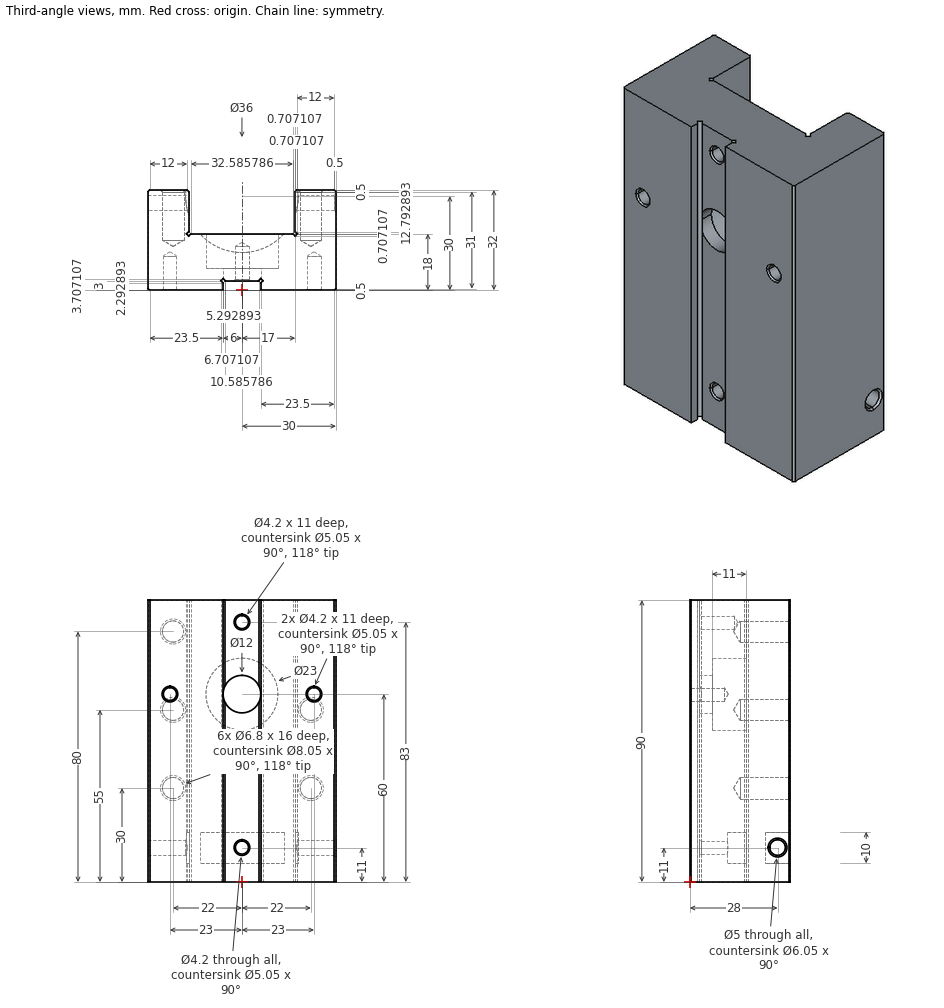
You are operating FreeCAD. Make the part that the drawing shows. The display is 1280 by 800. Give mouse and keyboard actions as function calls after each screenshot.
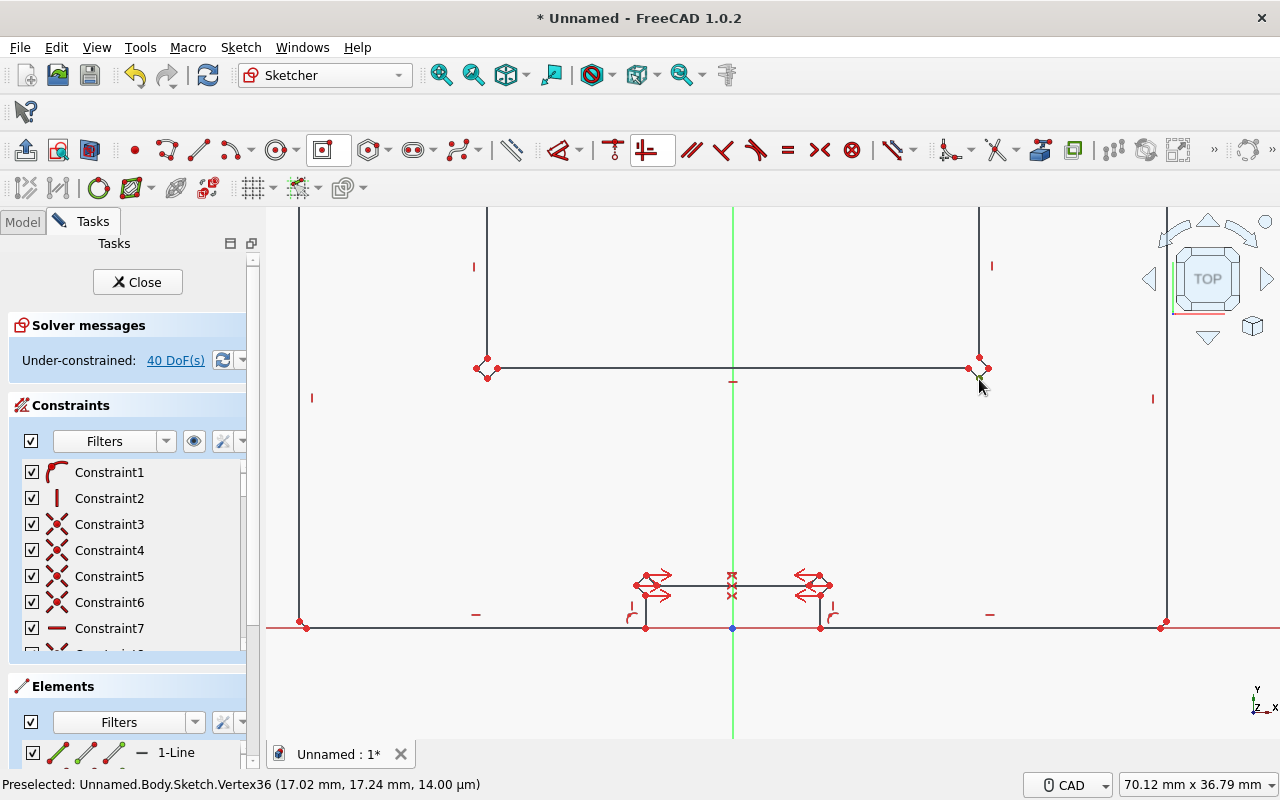
click(487, 379)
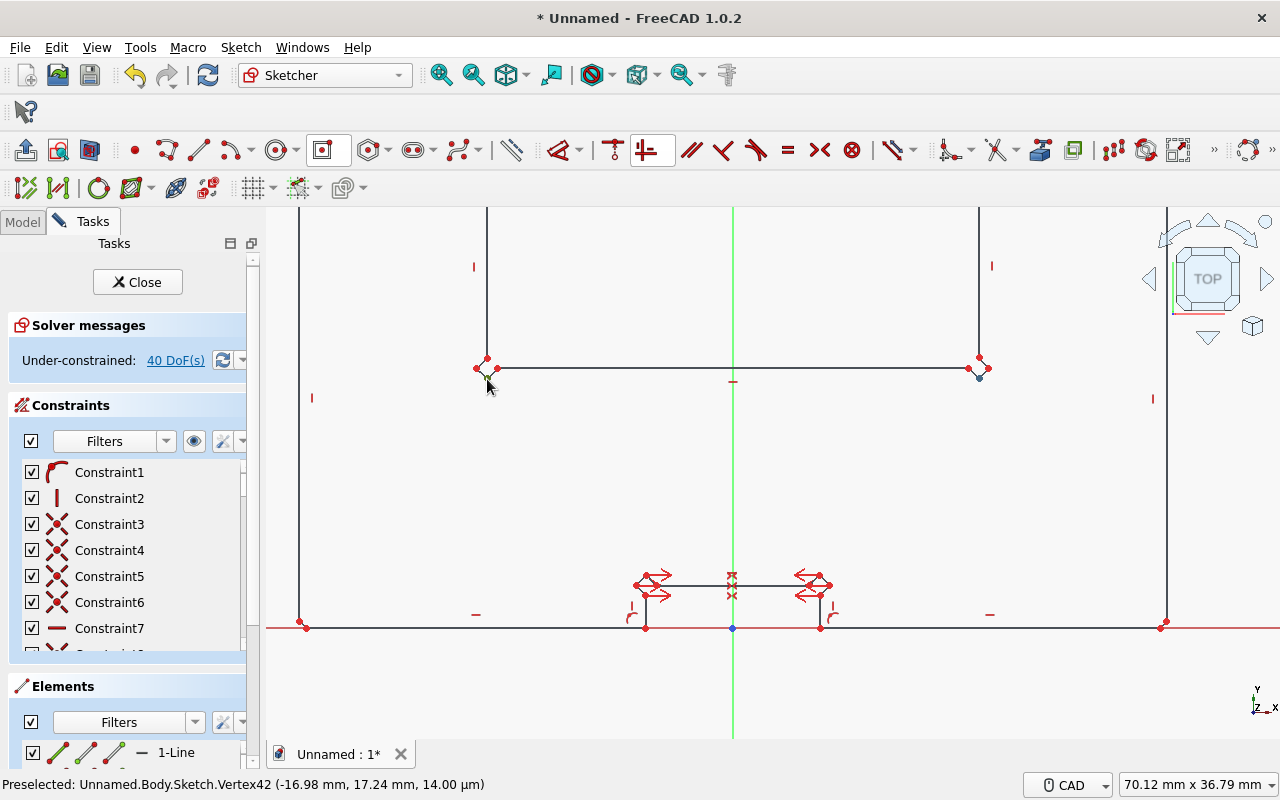
click(733, 677)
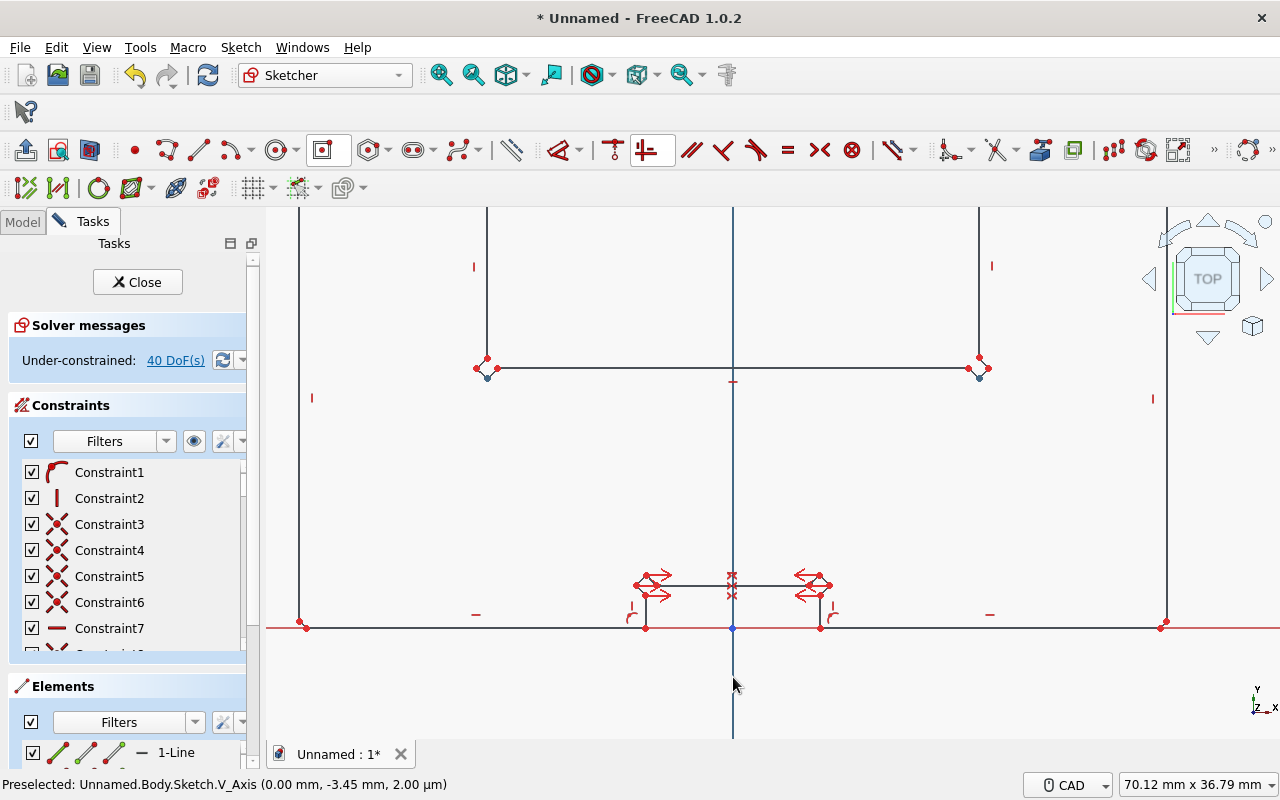
click(820, 150)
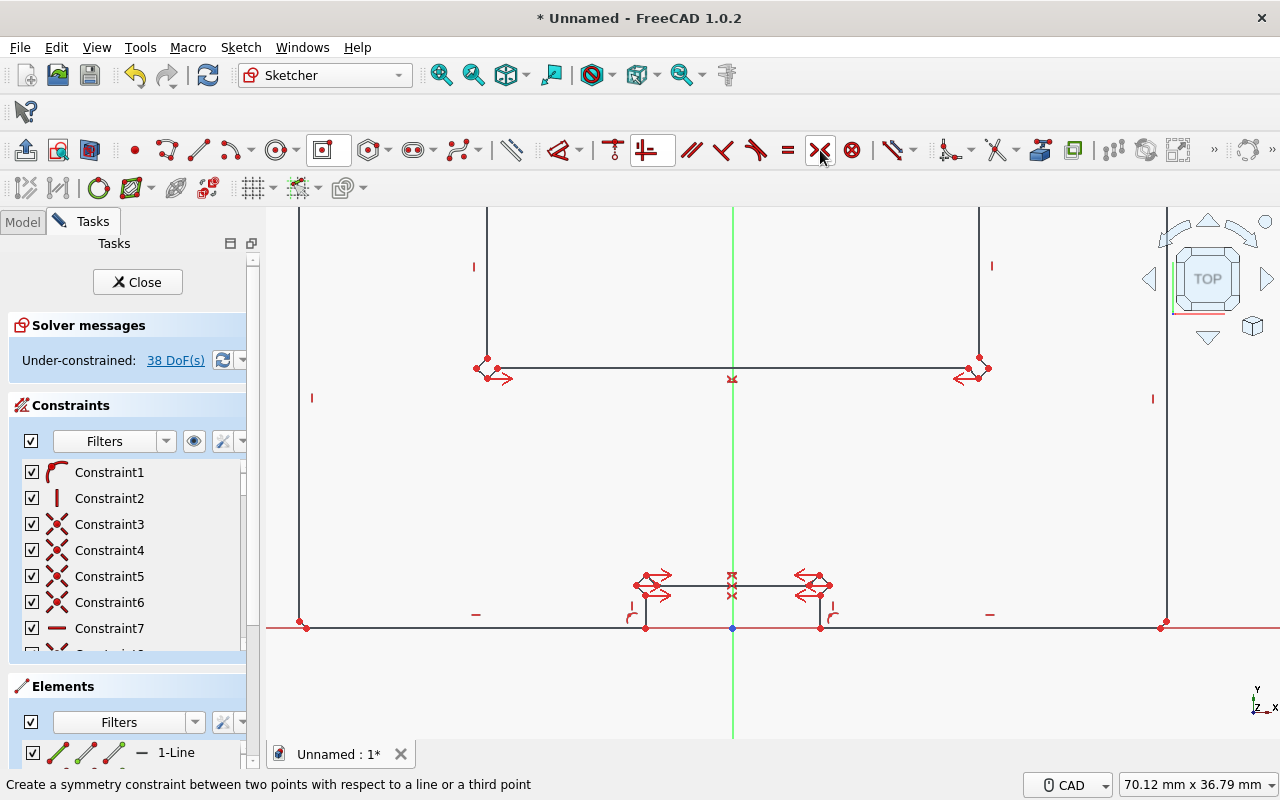
click(989, 368)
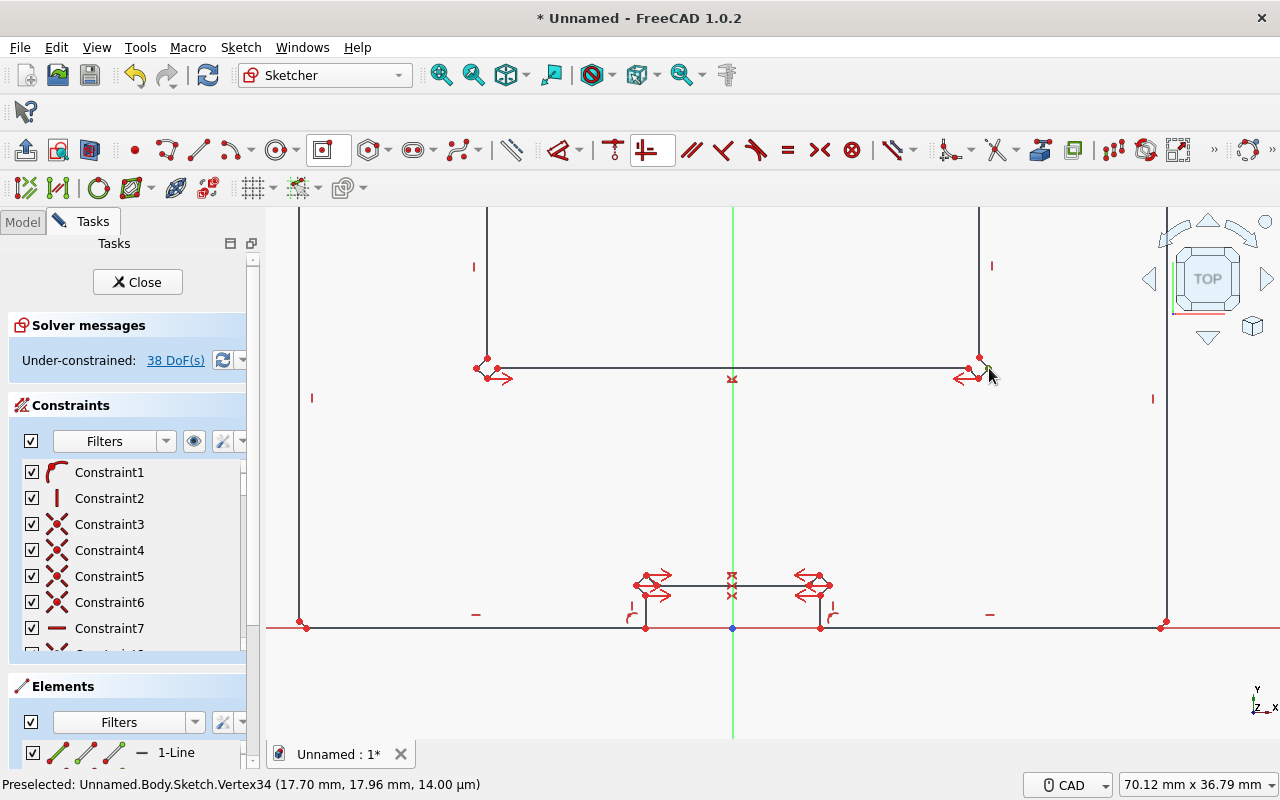
click(477, 369)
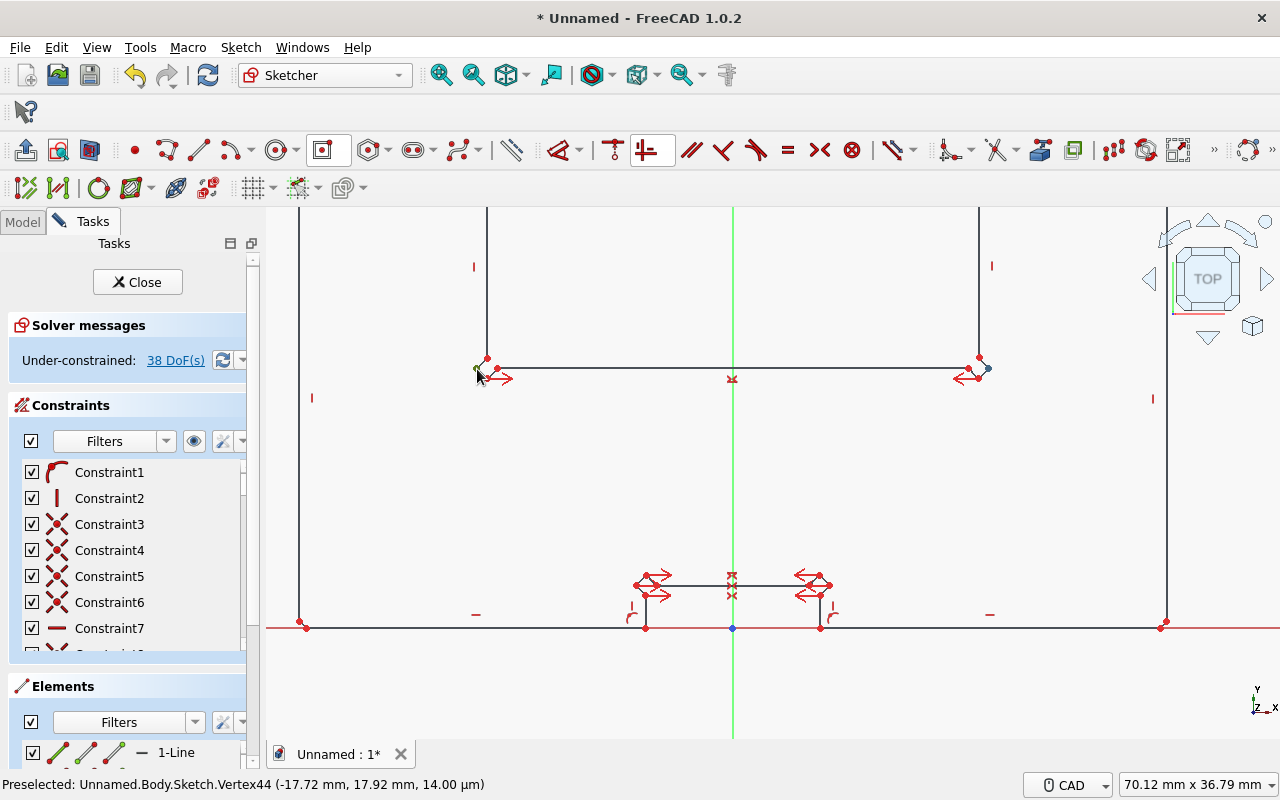
click(733, 677)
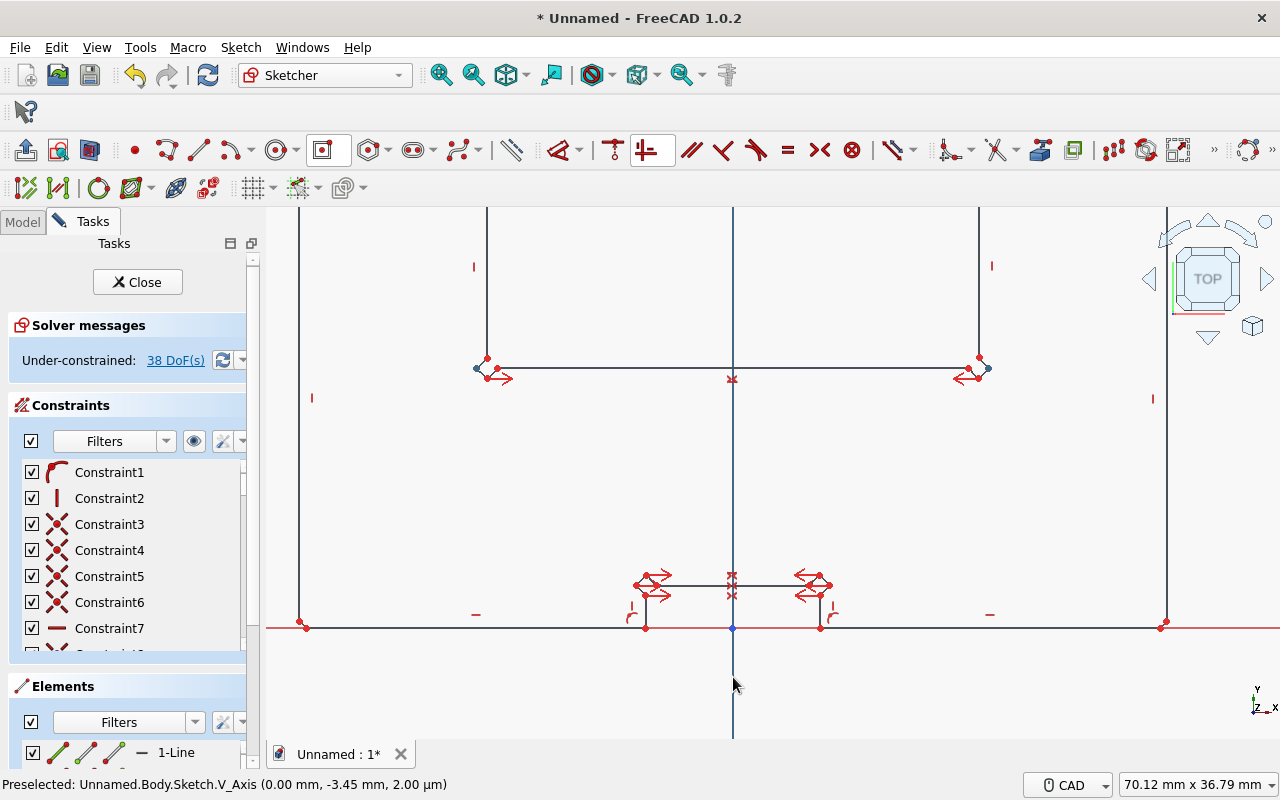
click(820, 150)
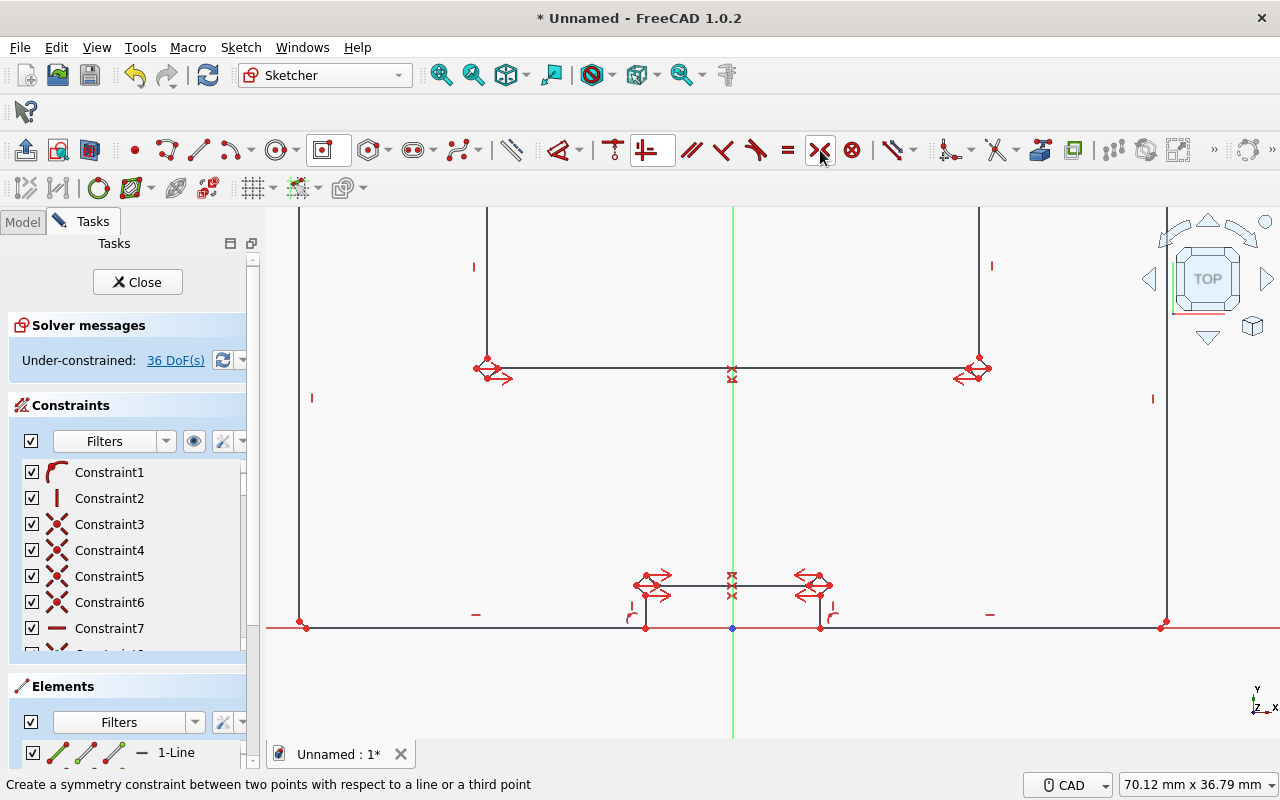
click(979, 358)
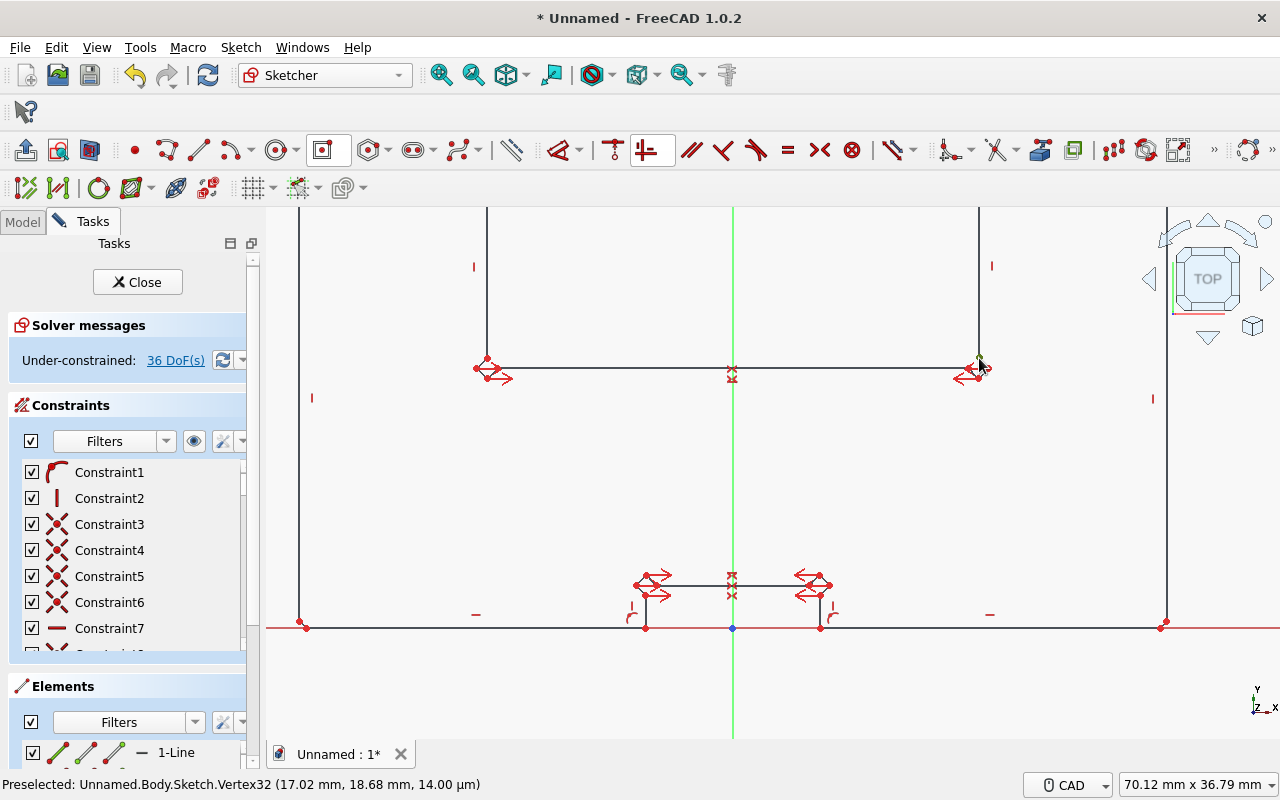
click(487, 358)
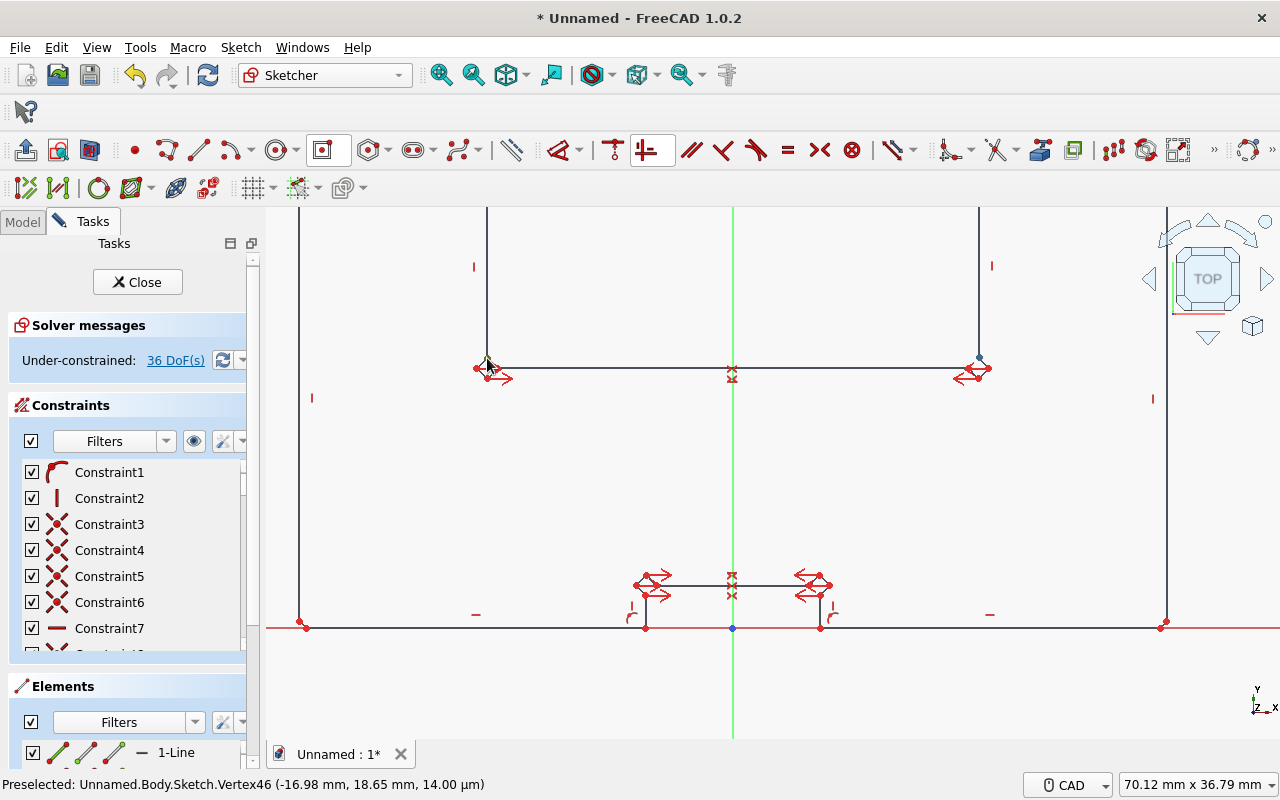
click(733, 677)